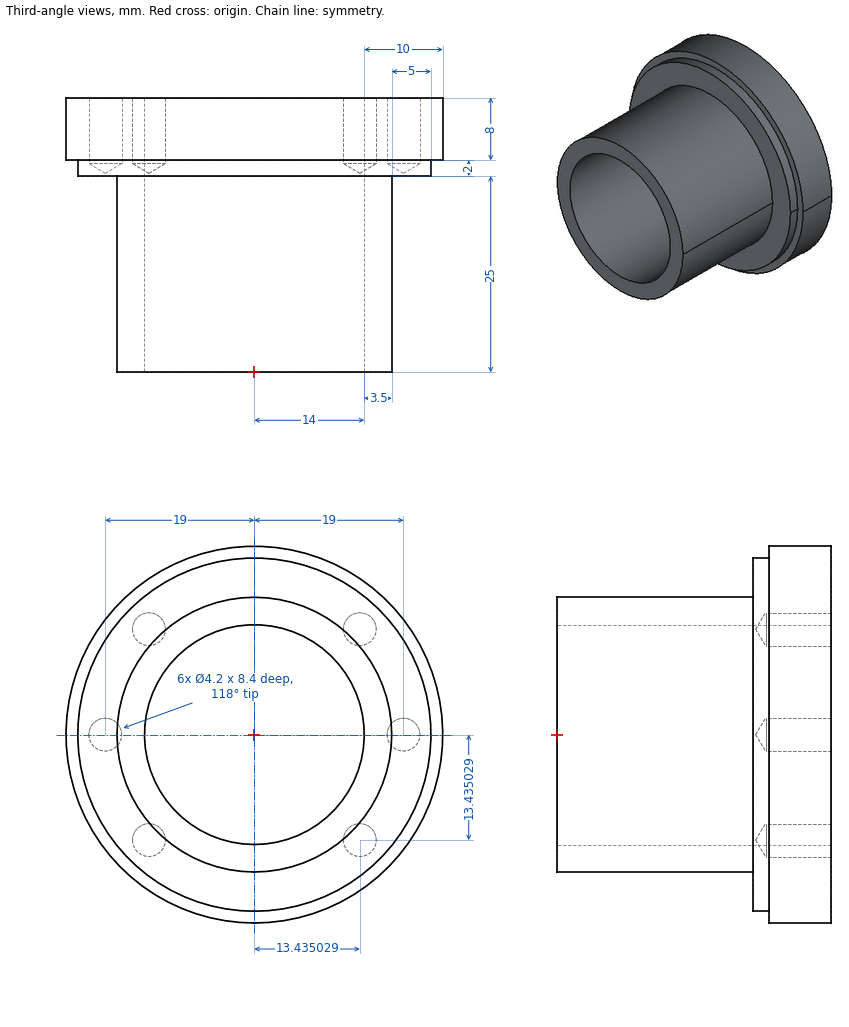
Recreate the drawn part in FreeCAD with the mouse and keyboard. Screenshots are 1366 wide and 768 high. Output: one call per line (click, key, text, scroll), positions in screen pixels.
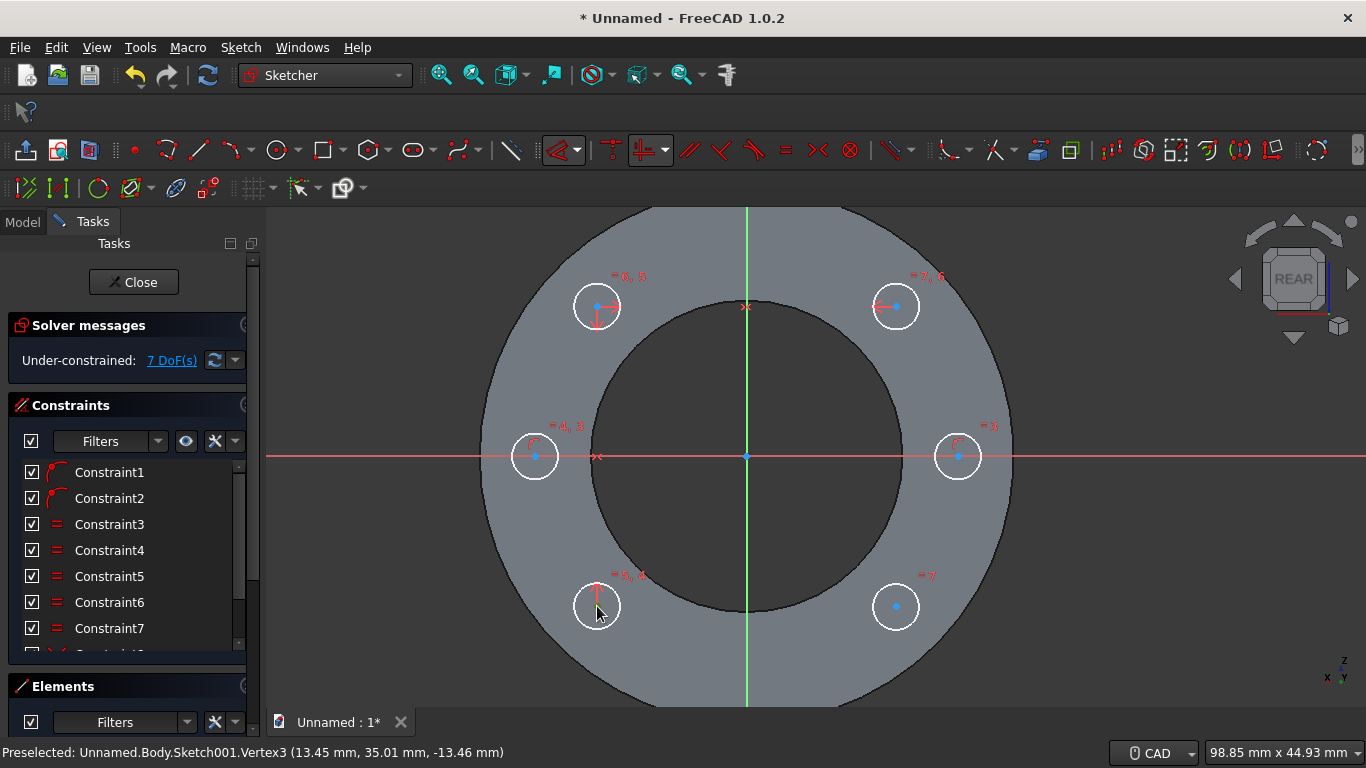
click(896, 607)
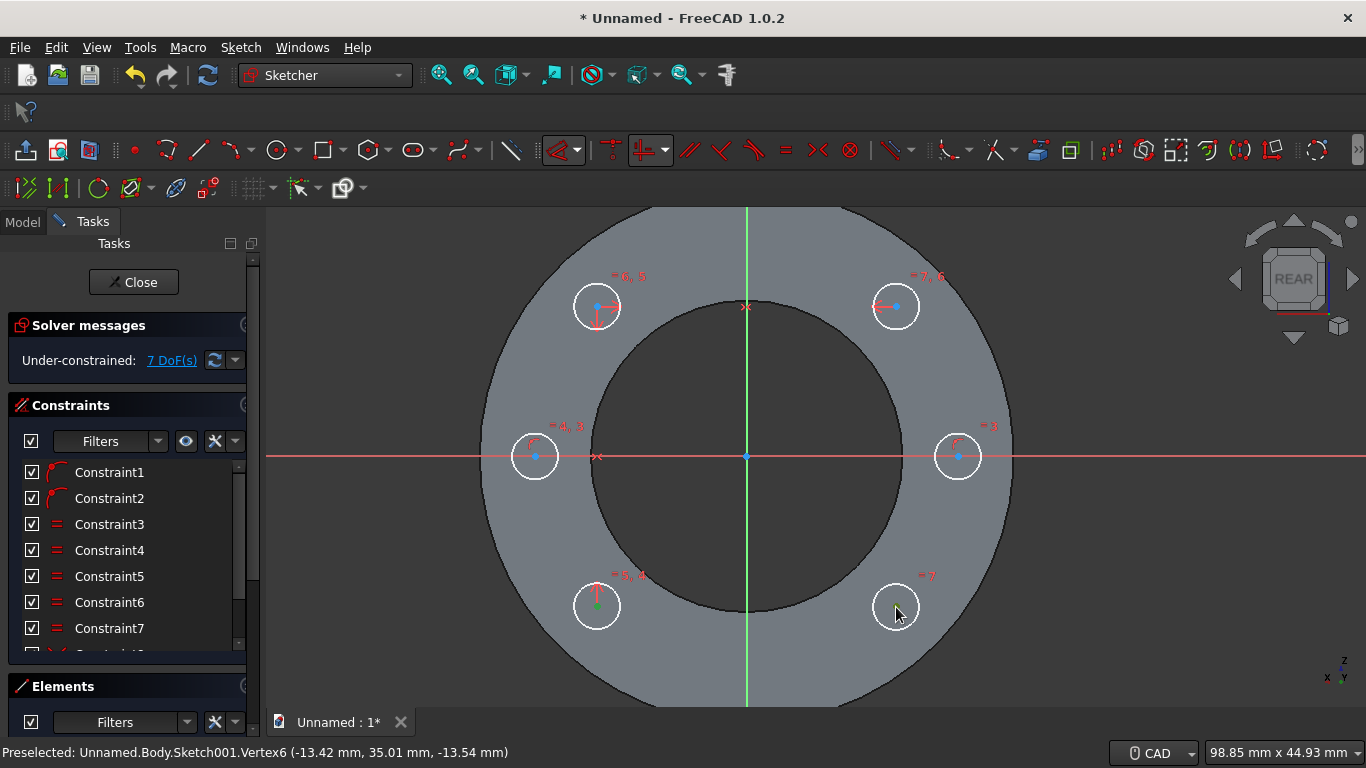
click(747, 647)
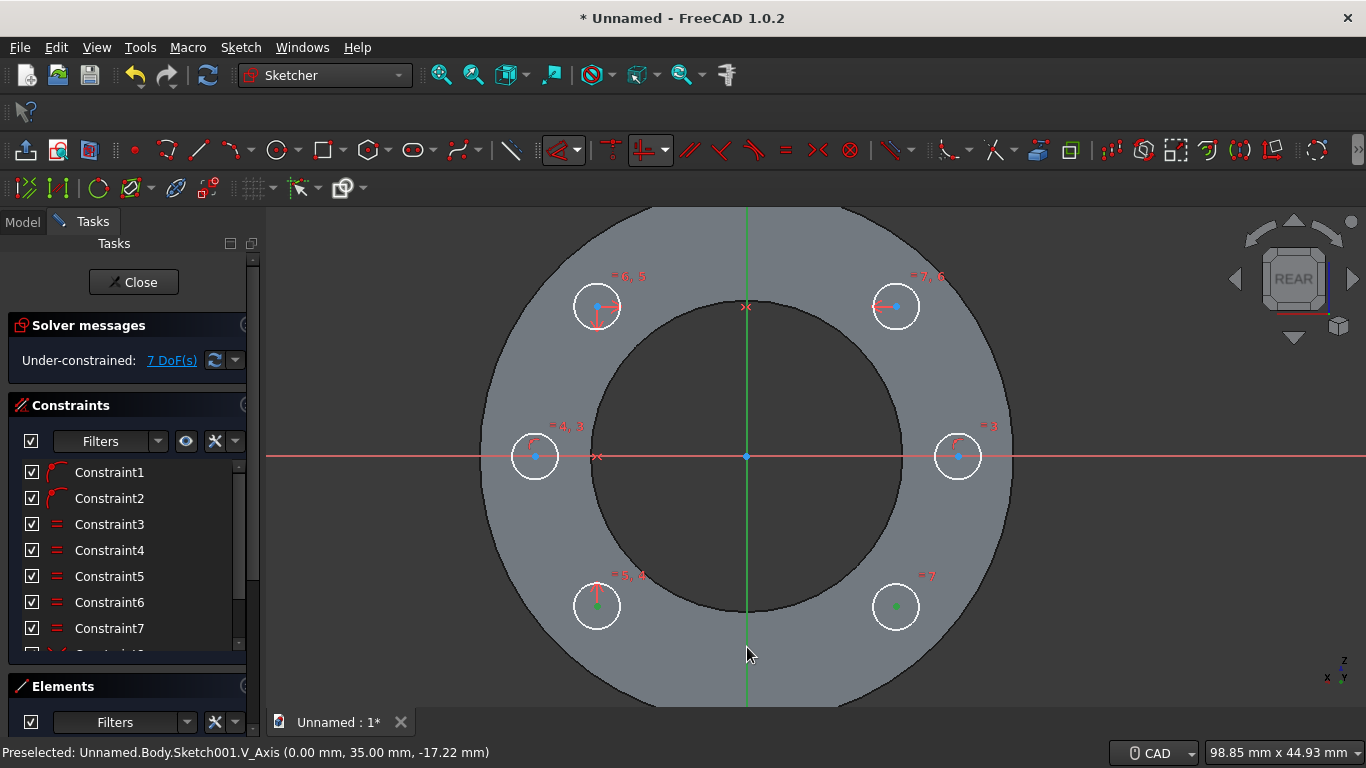
click(818, 150)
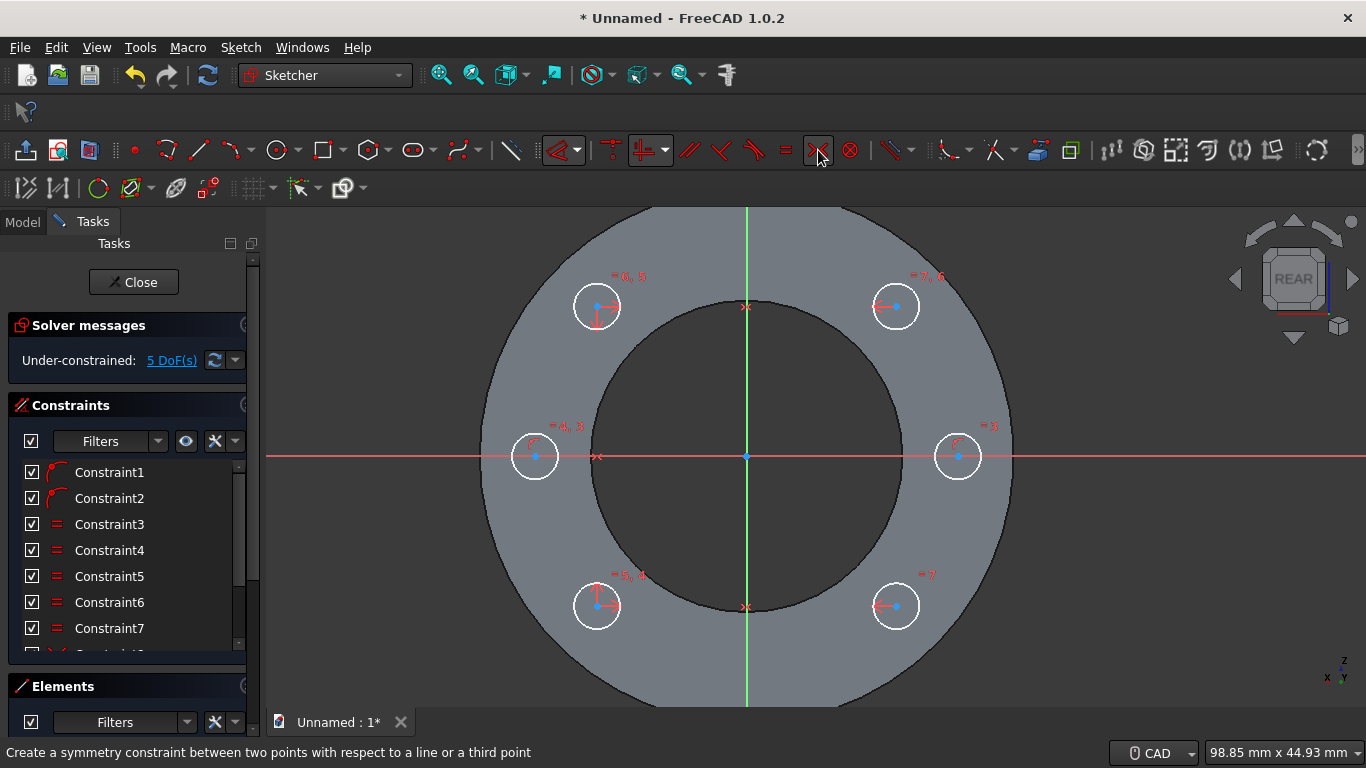
click(974, 440)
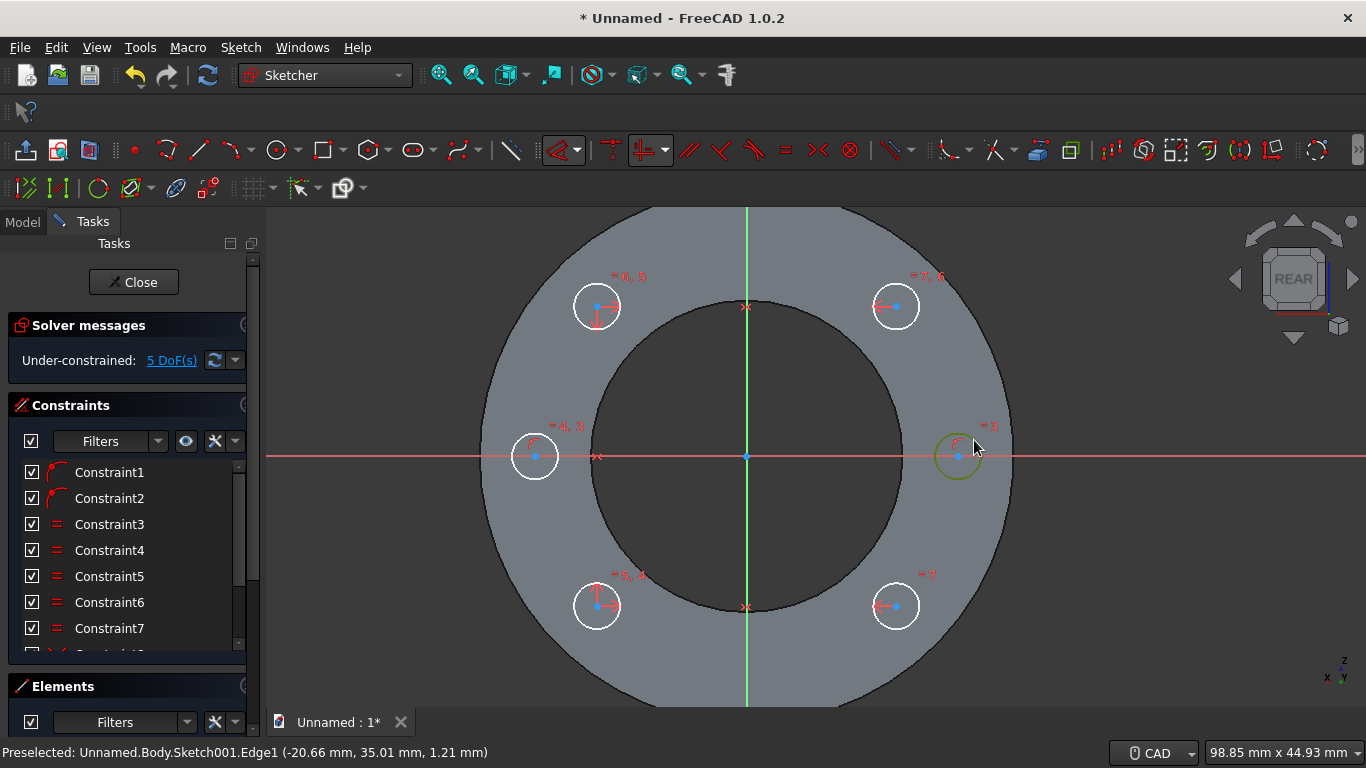
click(580, 150)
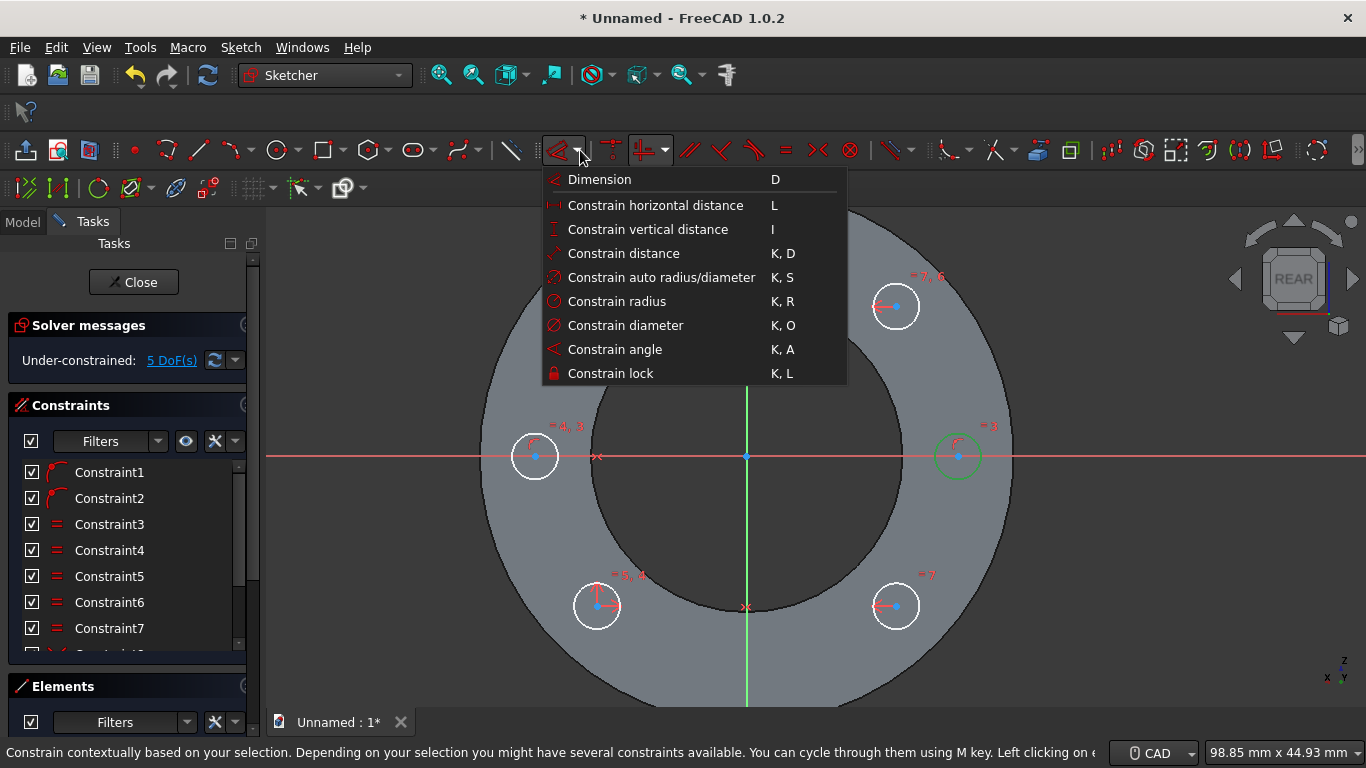
click(695, 325)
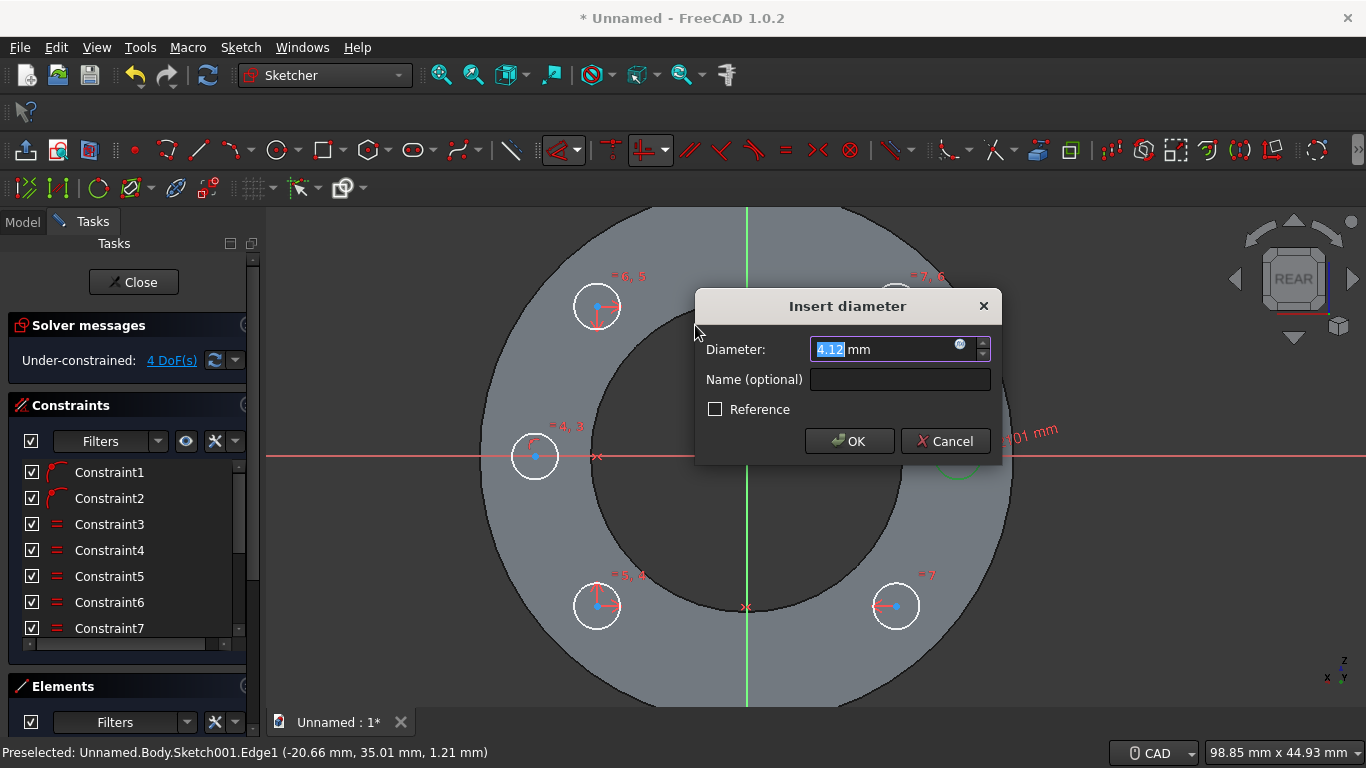
text(4.2)
key(Return)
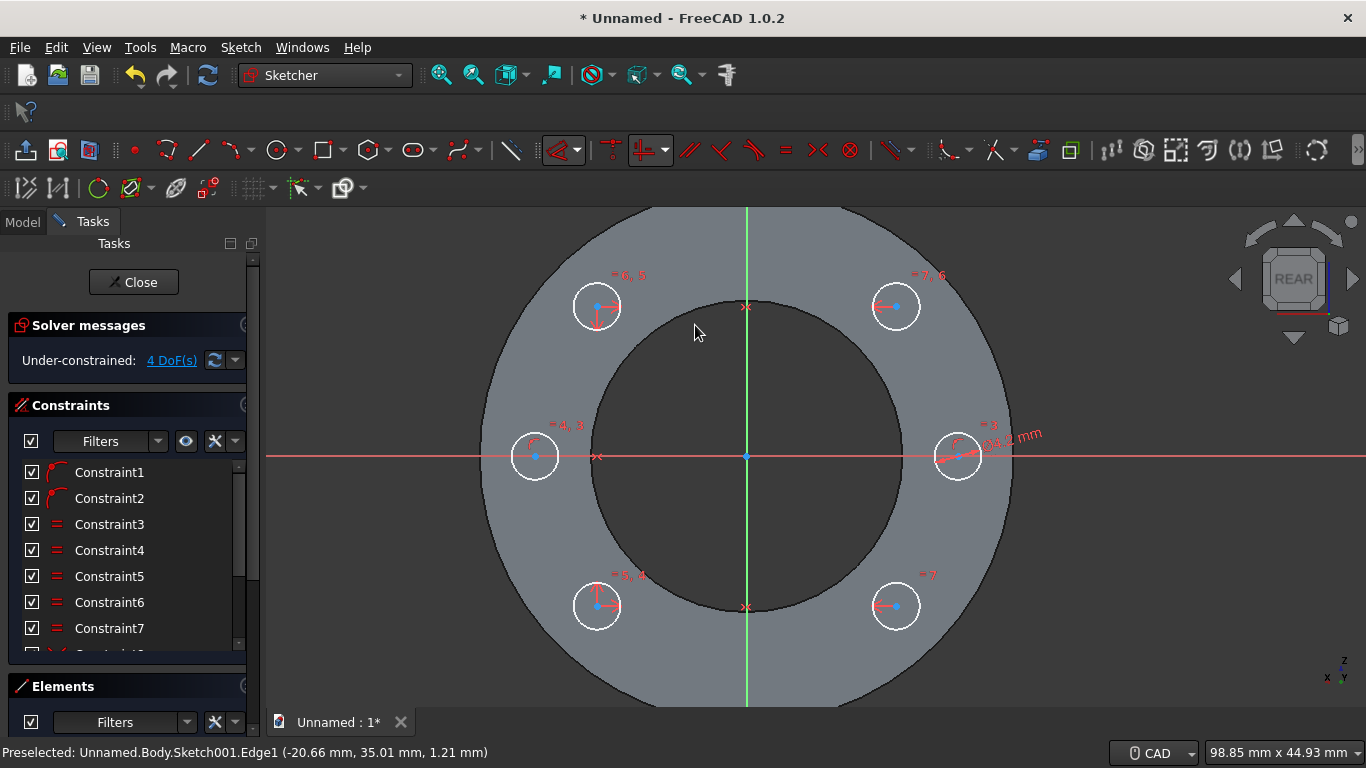
click(958, 456)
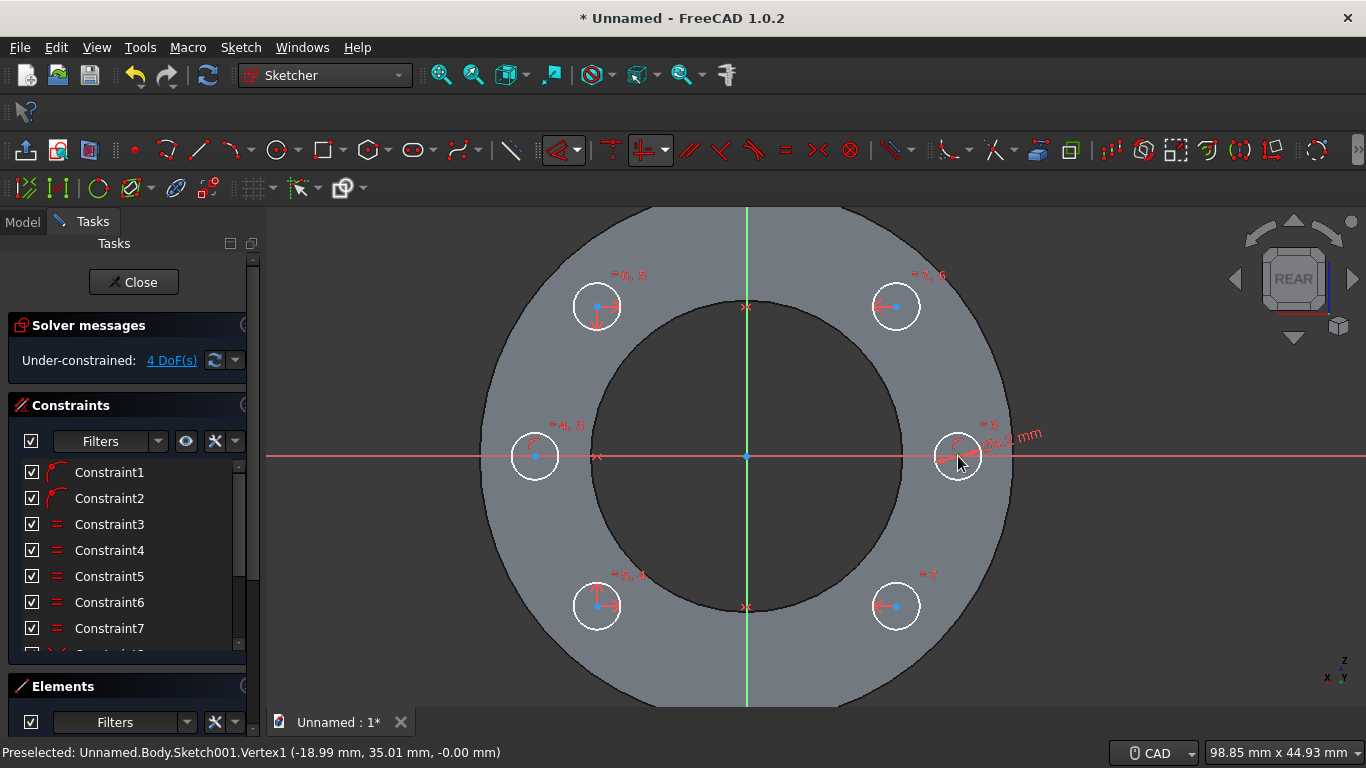
click(580, 150)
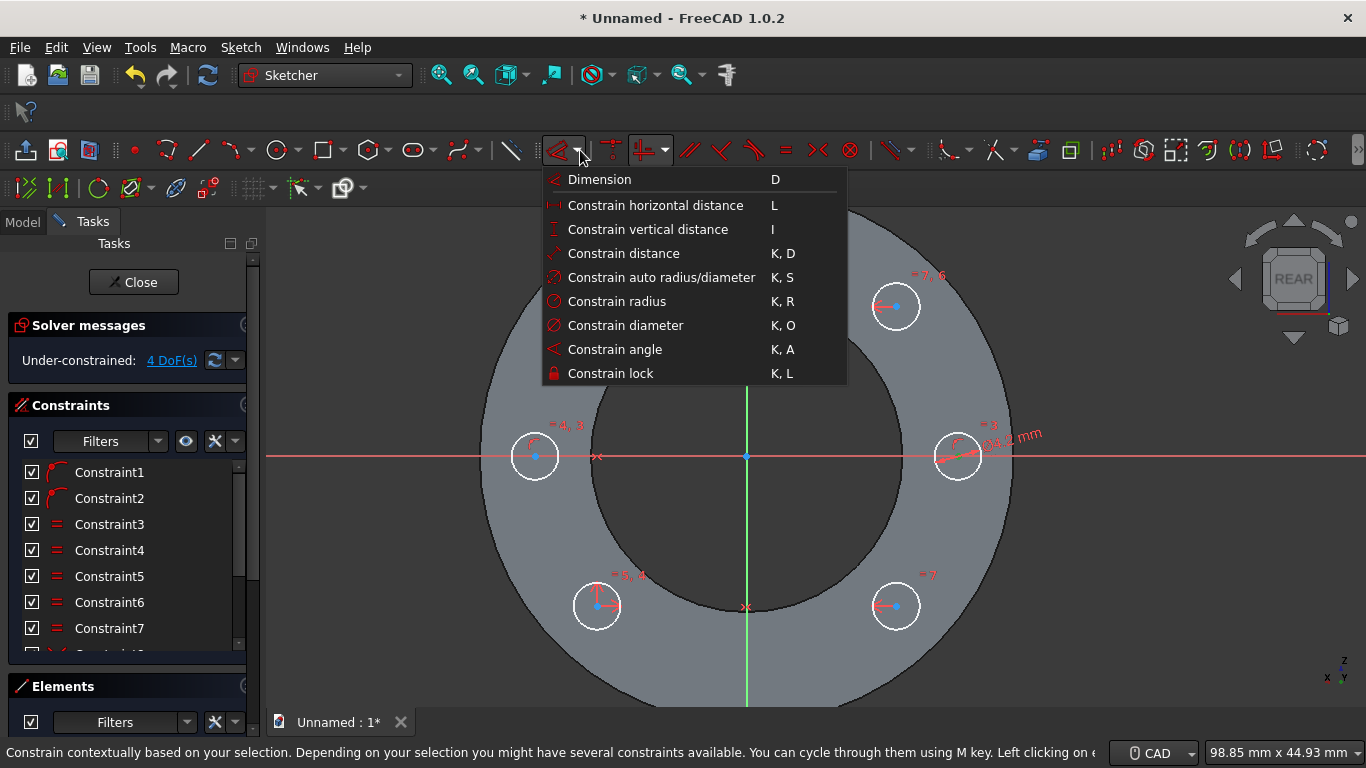
click(695, 205)